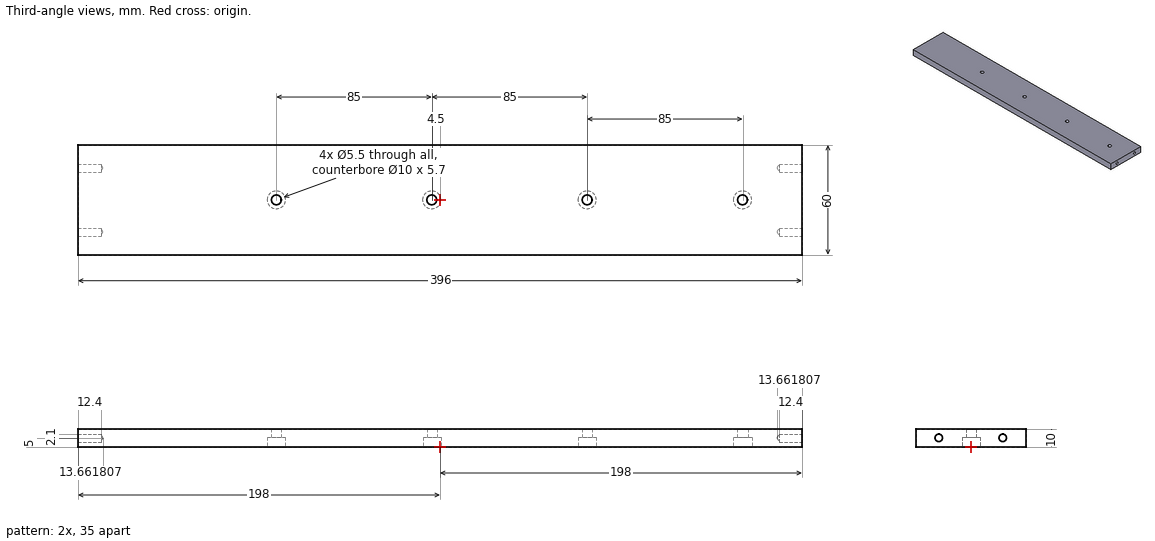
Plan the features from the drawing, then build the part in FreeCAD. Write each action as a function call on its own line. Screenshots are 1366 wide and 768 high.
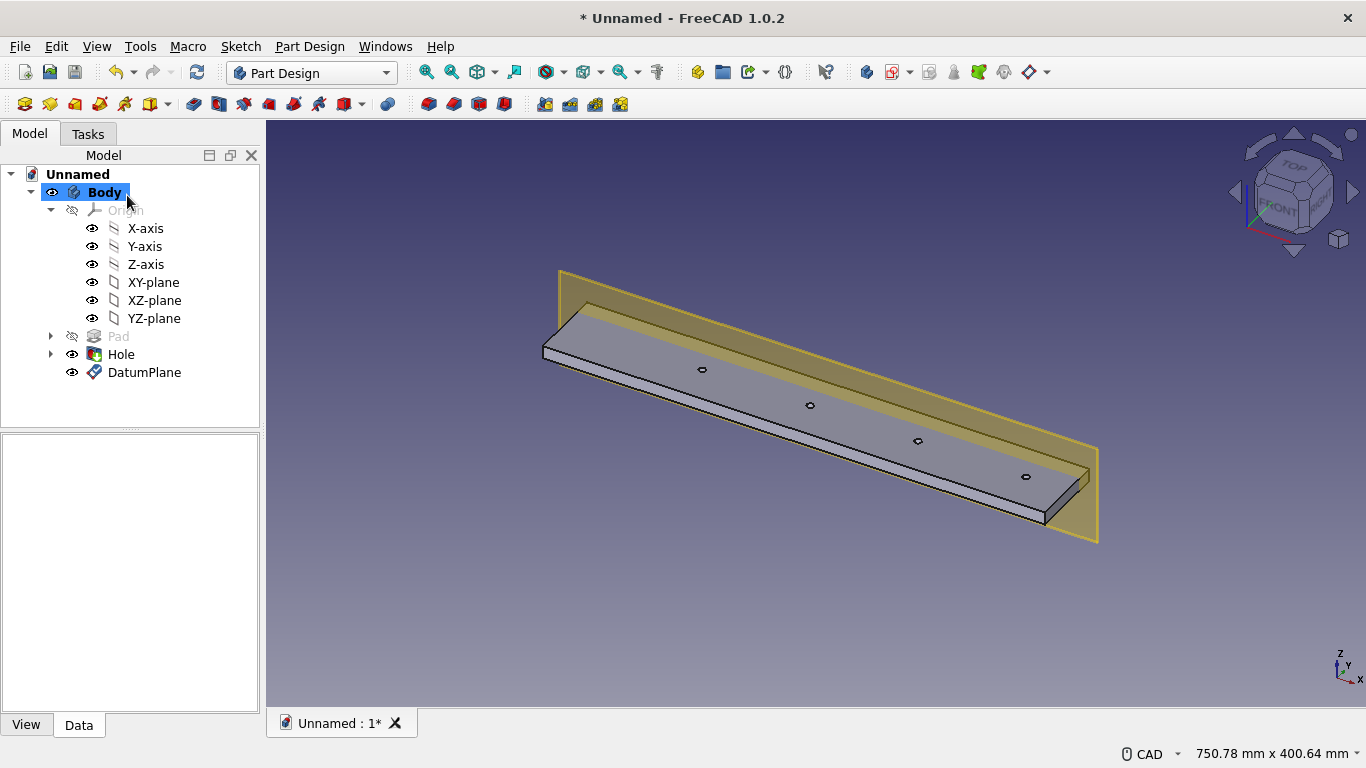
click(117, 372)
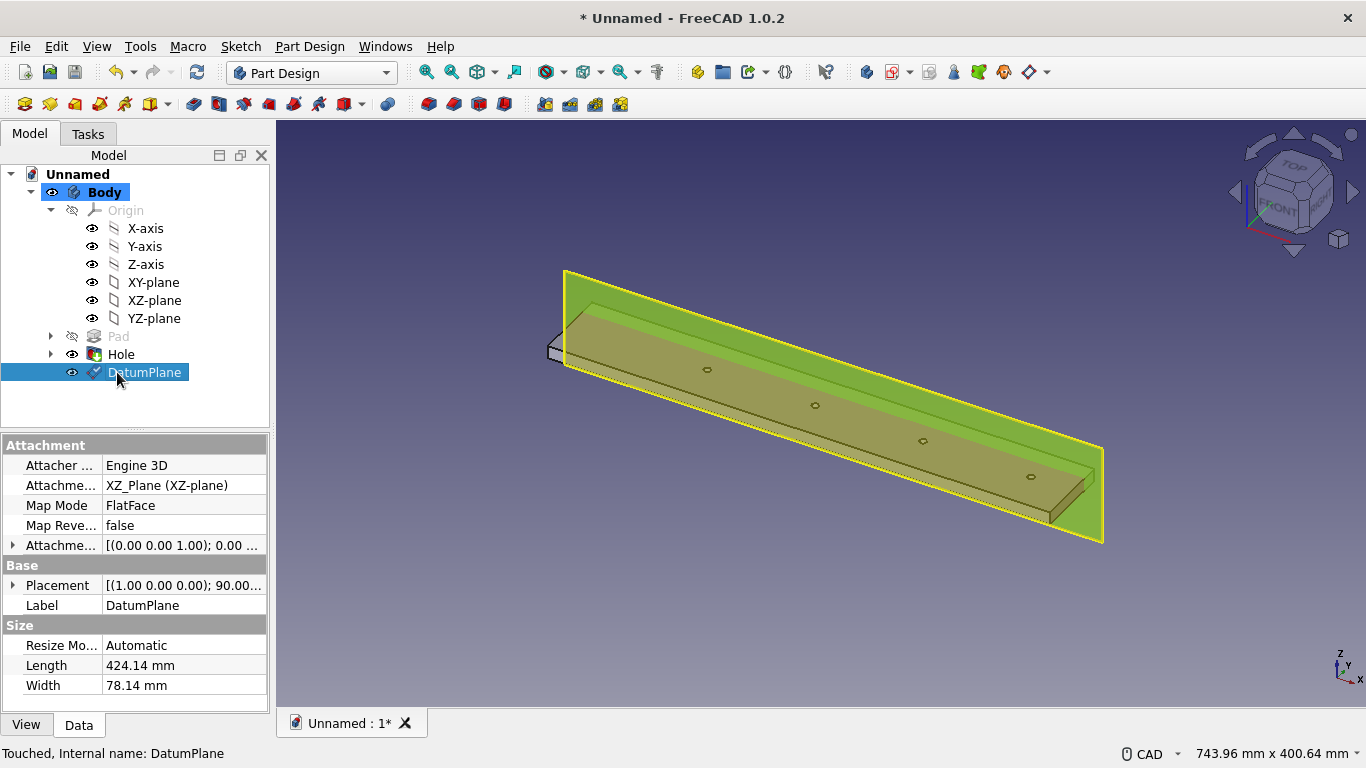
click(892, 72)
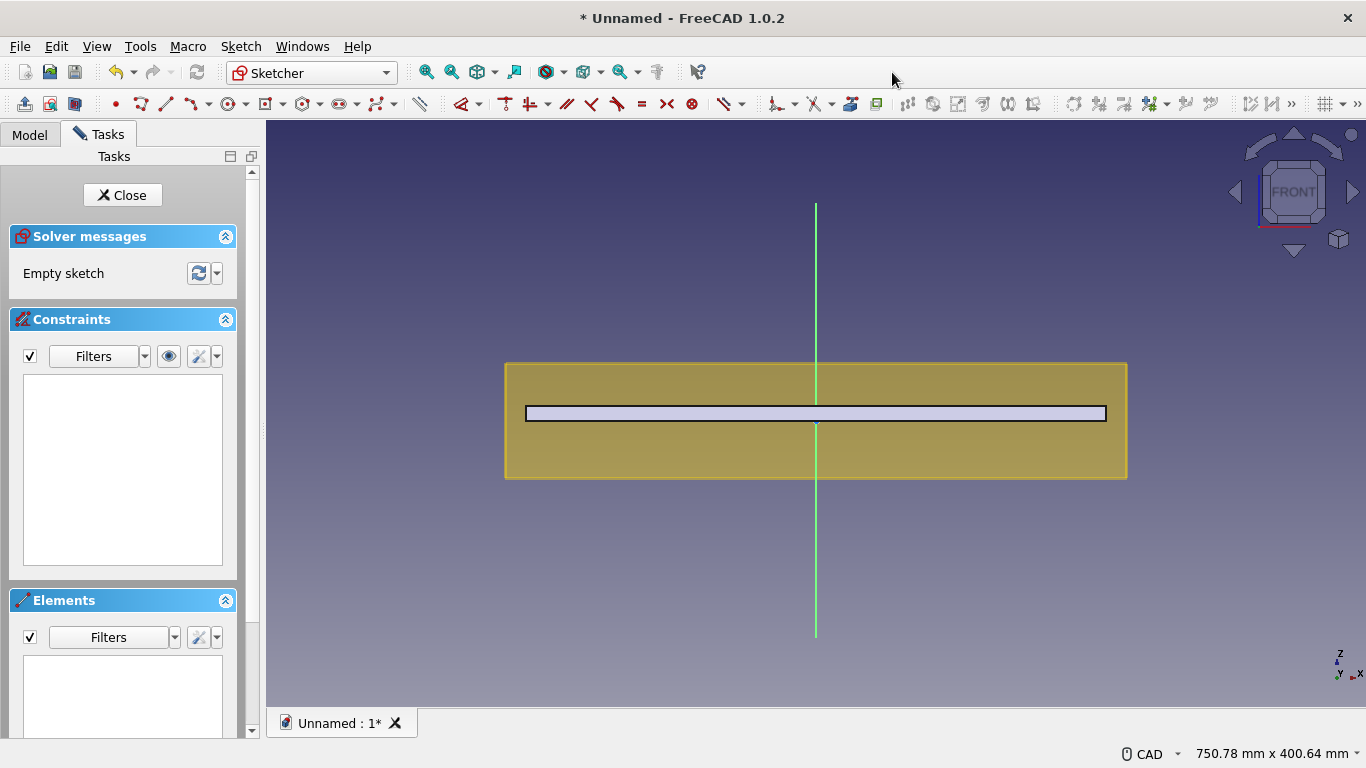
key(q)
key(s)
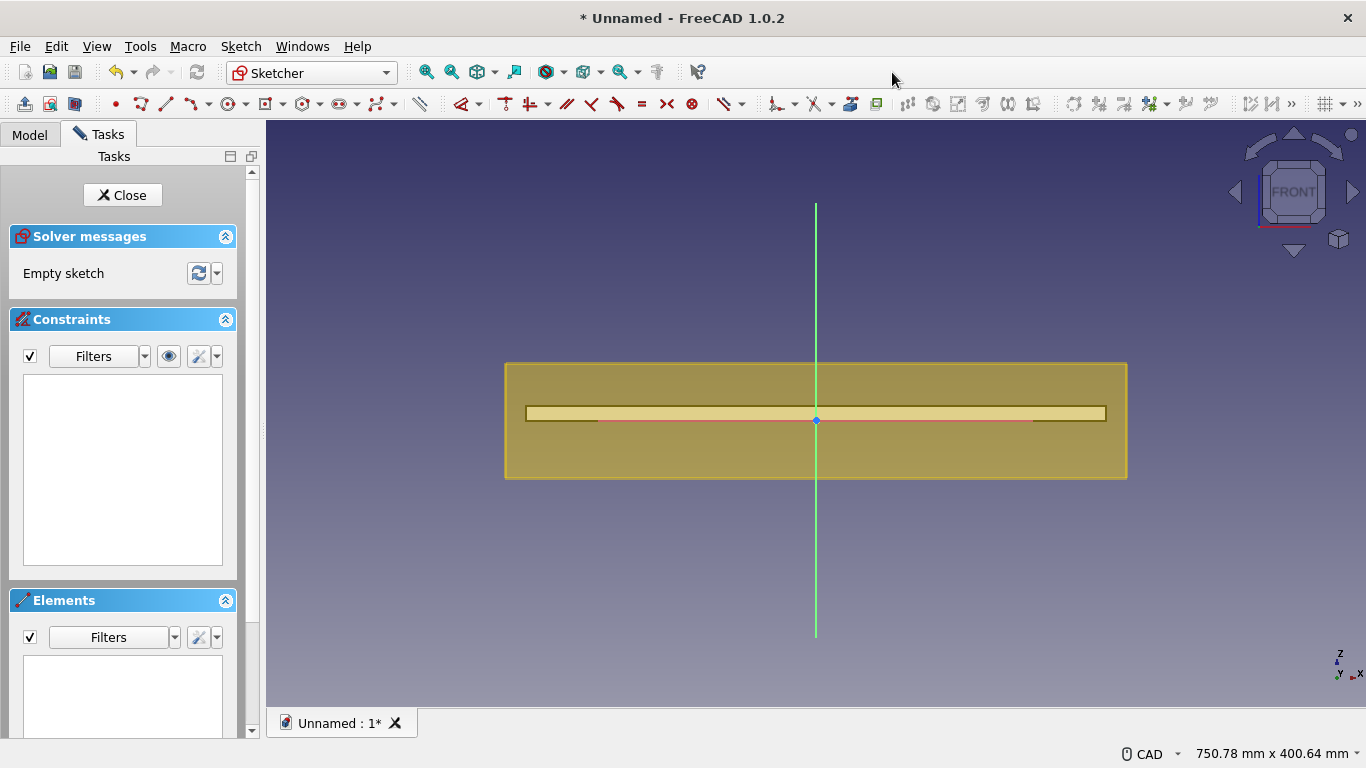
scroll(529, 412, up, 15)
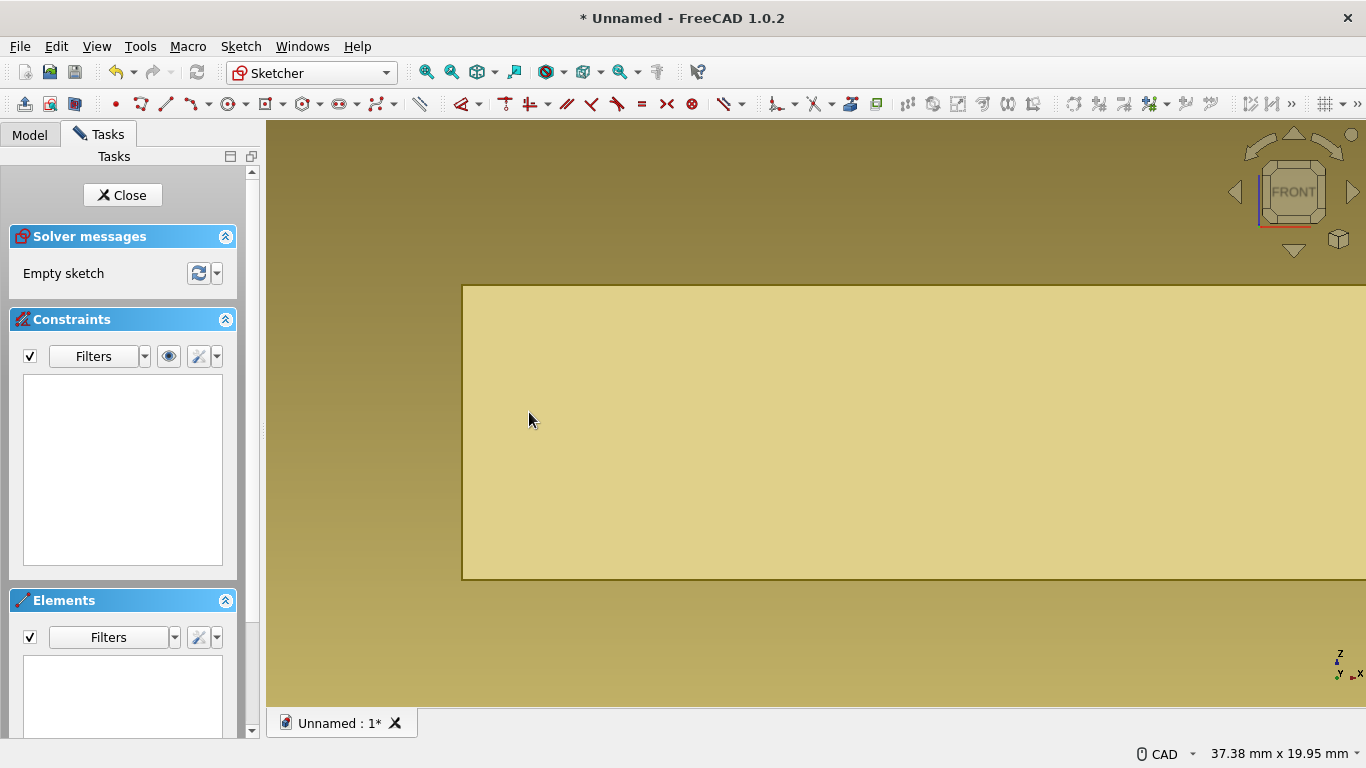
click(141, 104)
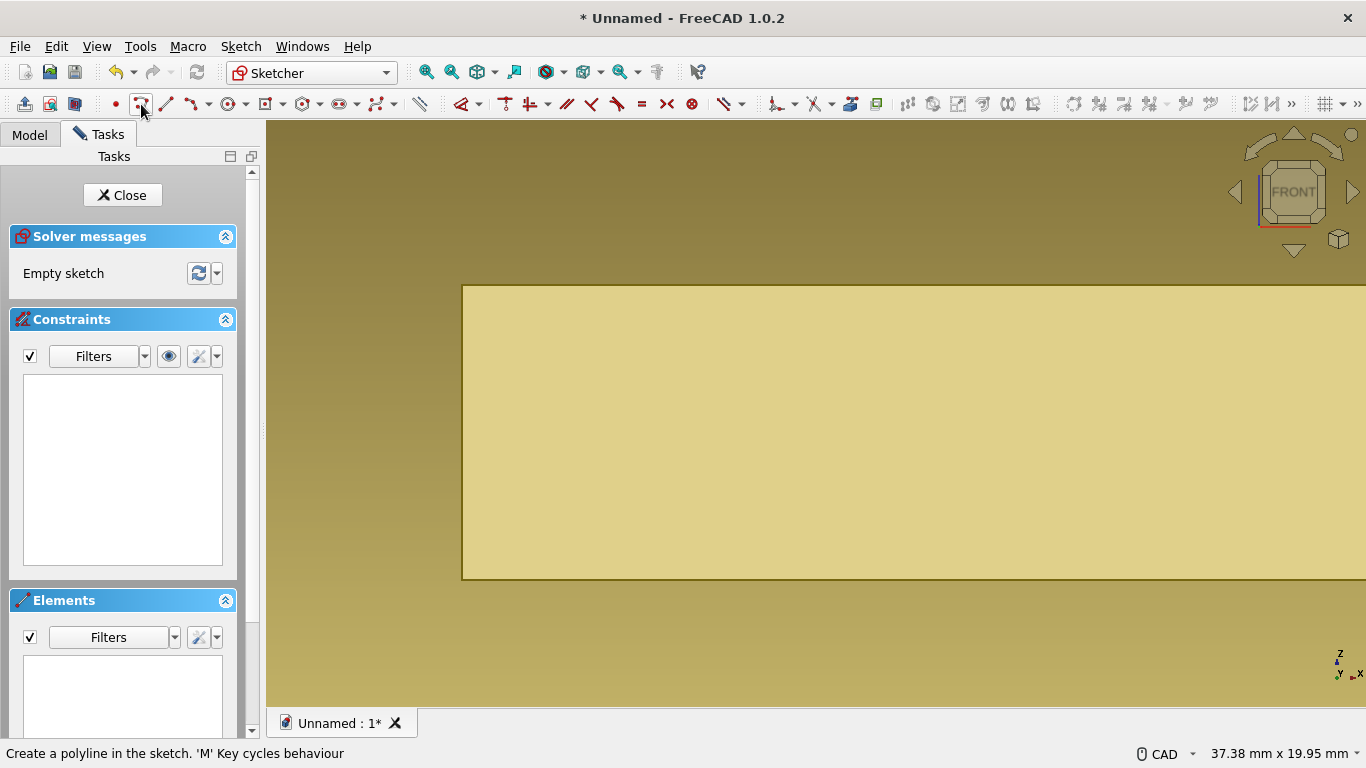
click(864, 433)
click(462, 433)
click(462, 371)
click(827, 371)
click(864, 434)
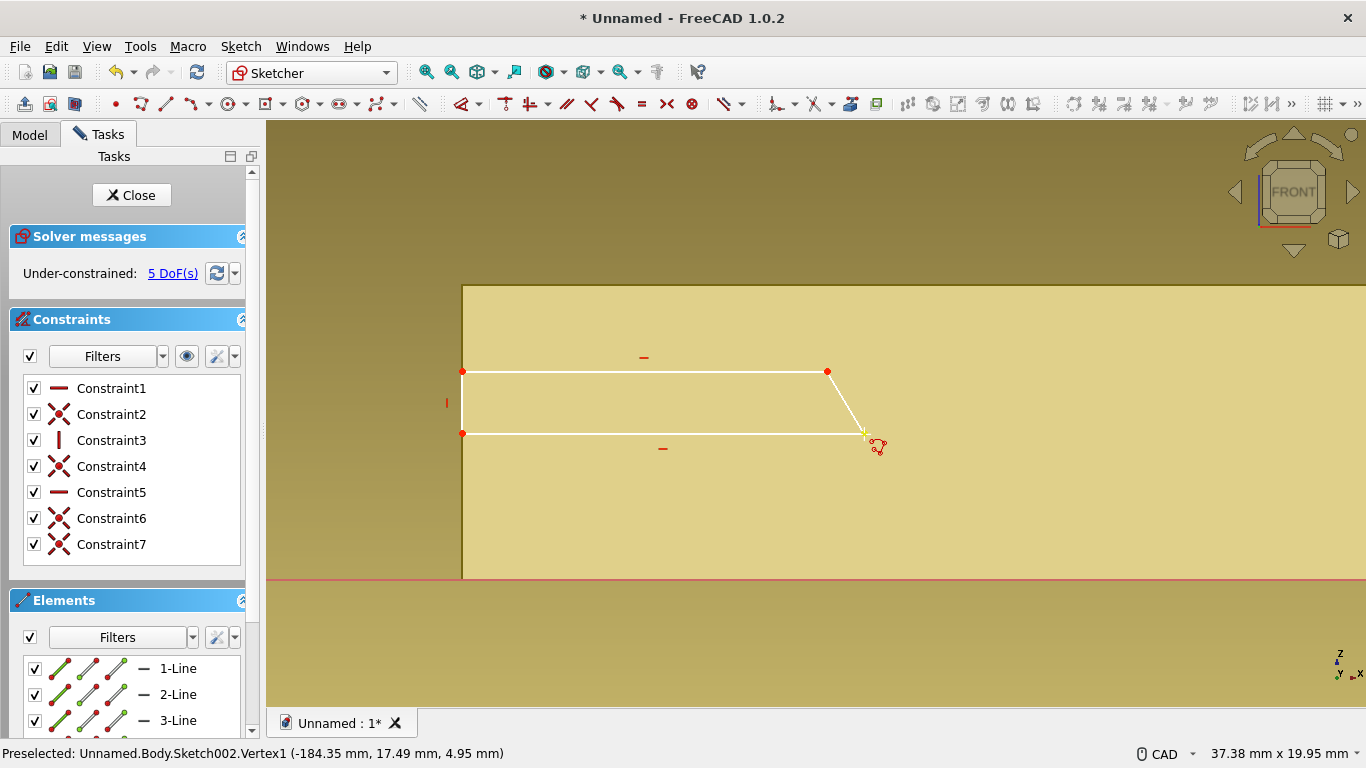
click(166, 104)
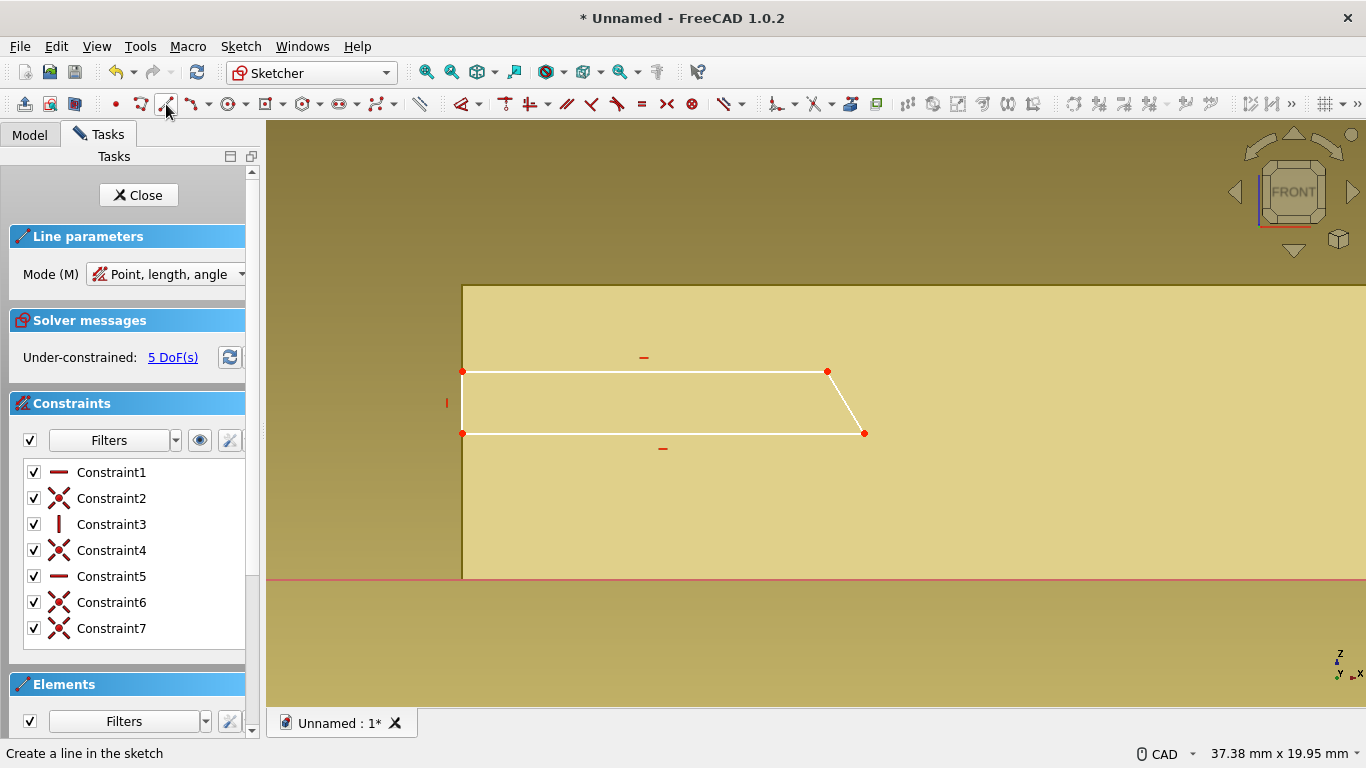
click(904, 433)
click(1025, 433)
key(Escape)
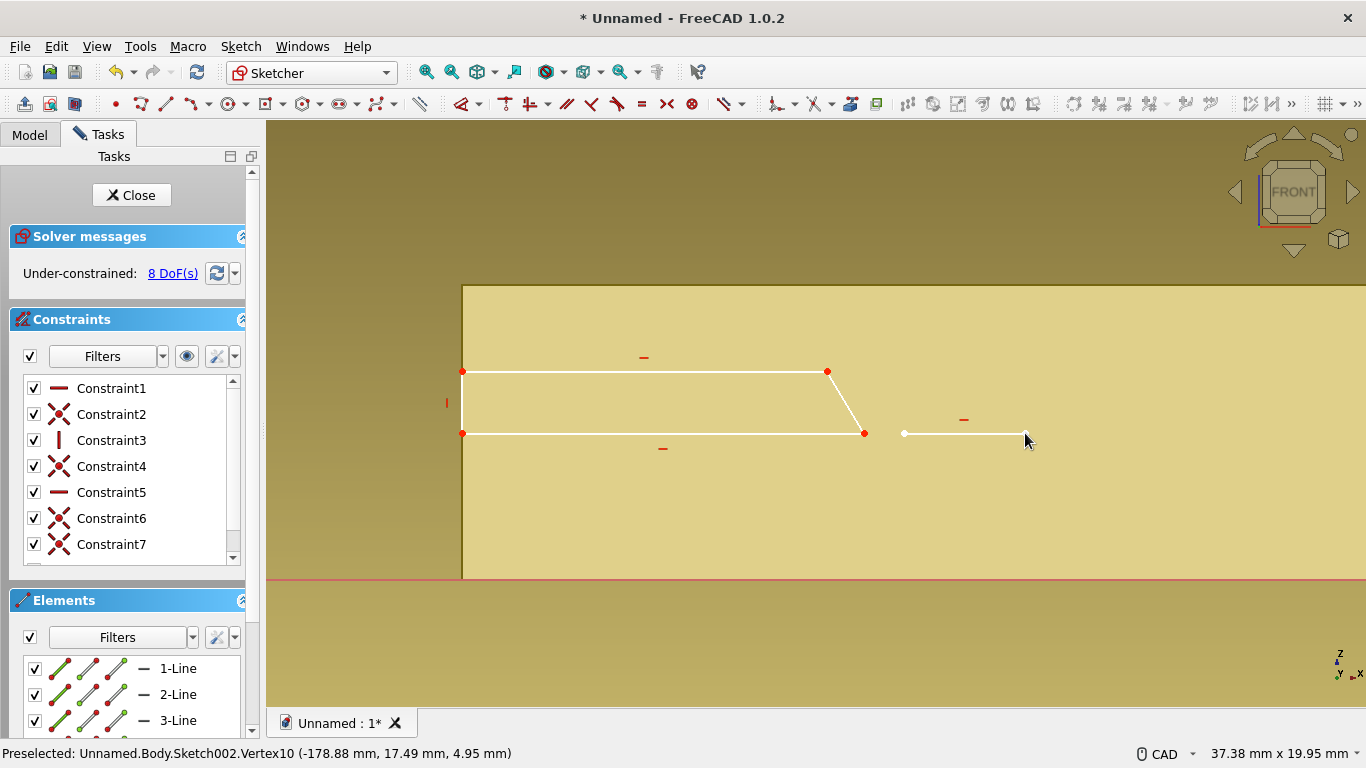
click(940, 434)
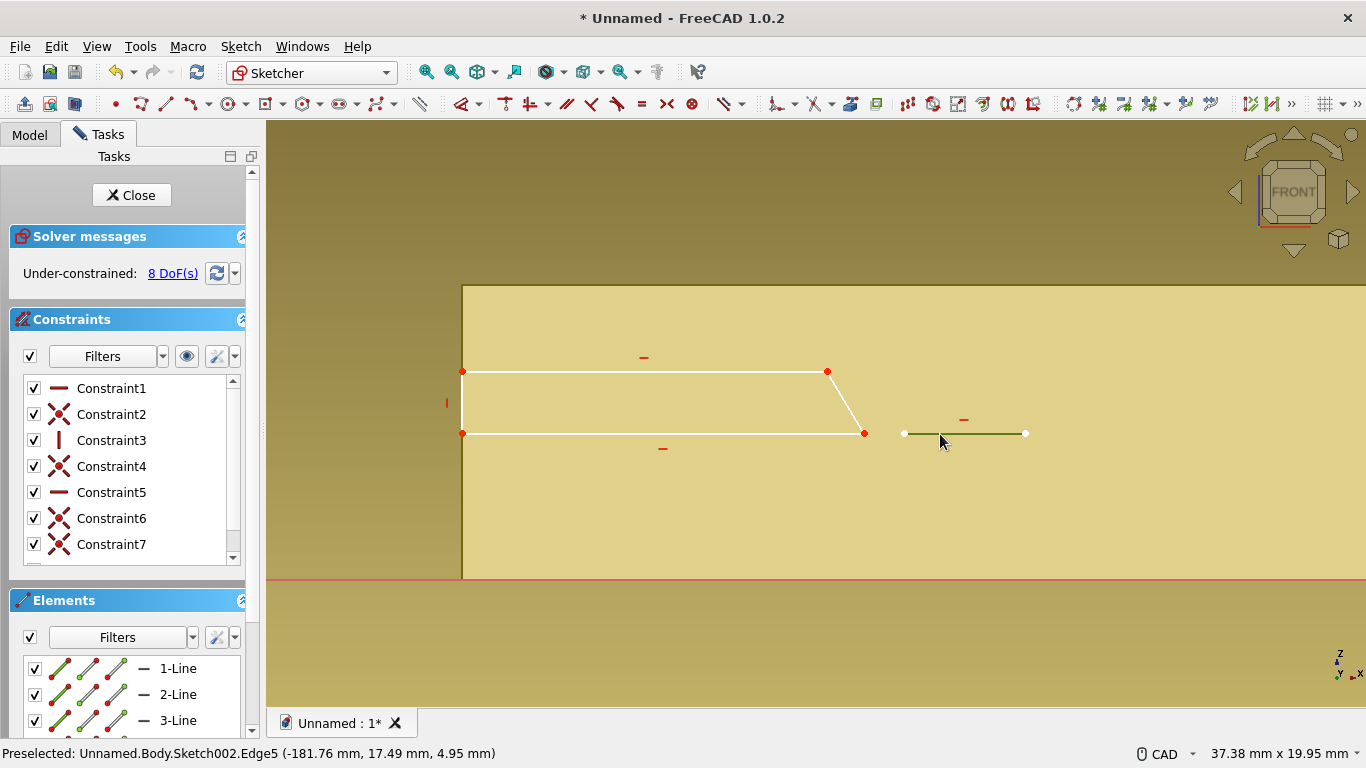
click(420, 104)